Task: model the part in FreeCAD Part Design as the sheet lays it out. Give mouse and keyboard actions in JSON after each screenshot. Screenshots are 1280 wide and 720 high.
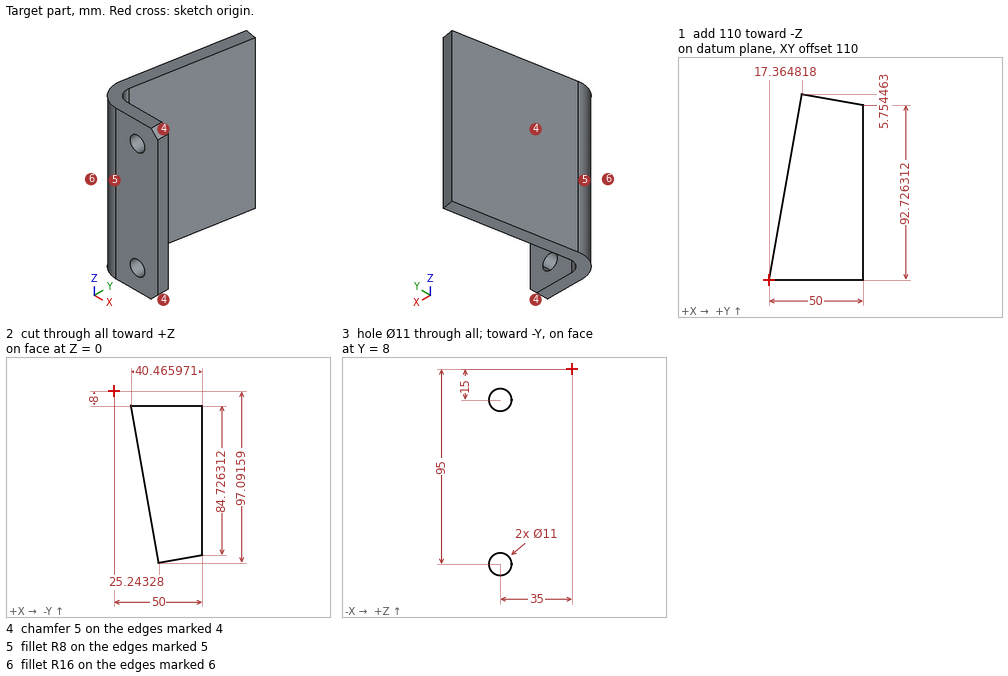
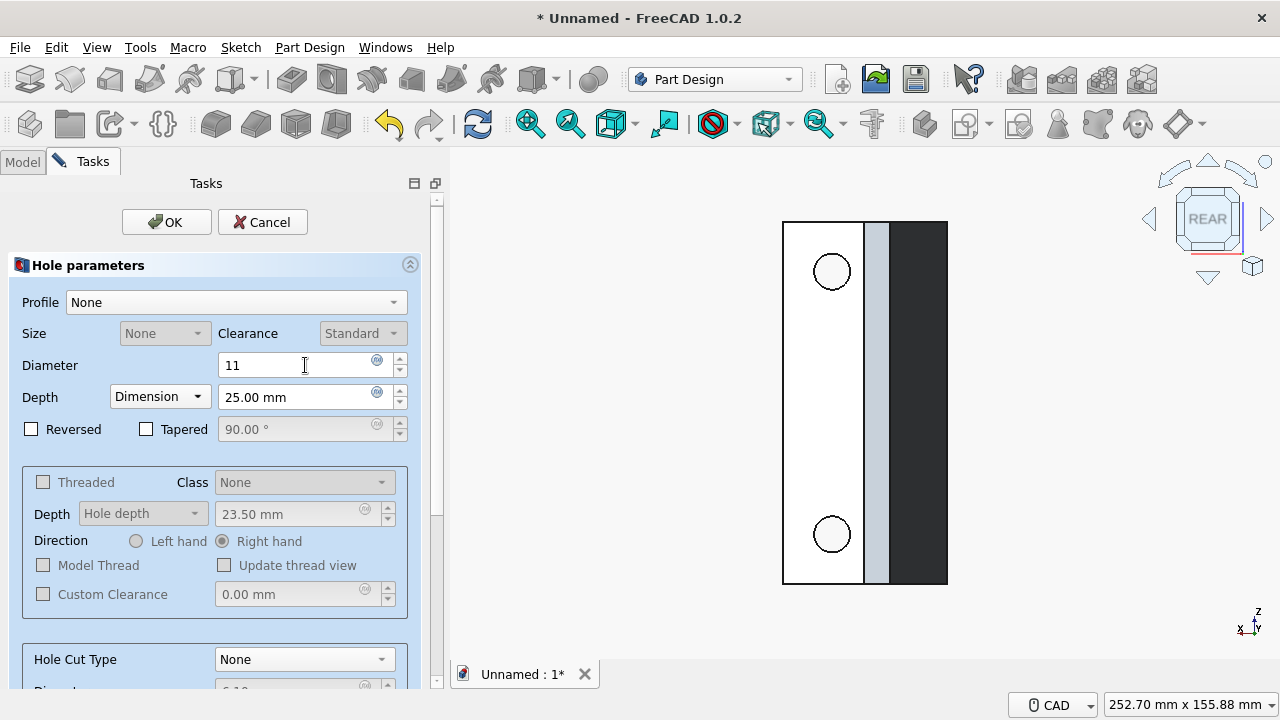
{"action": "left_click", "coordinate": [161, 396]}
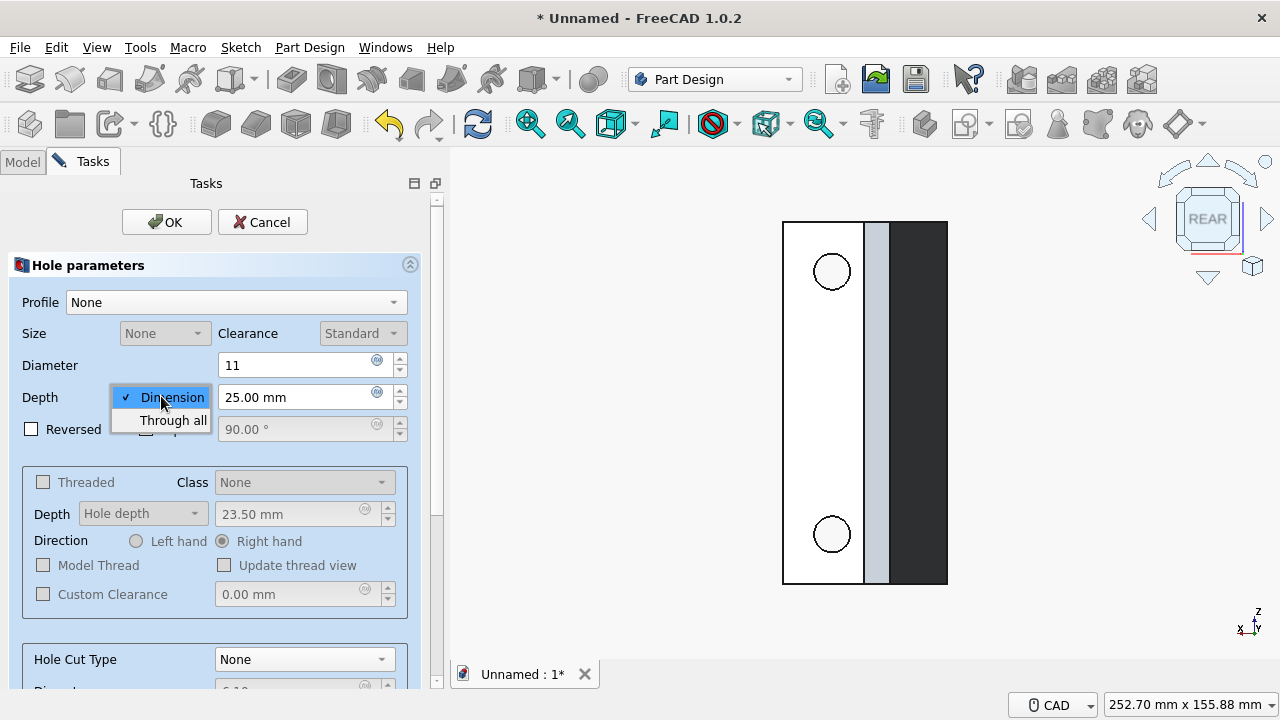
{"action": "left_click", "coordinate": [160, 420]}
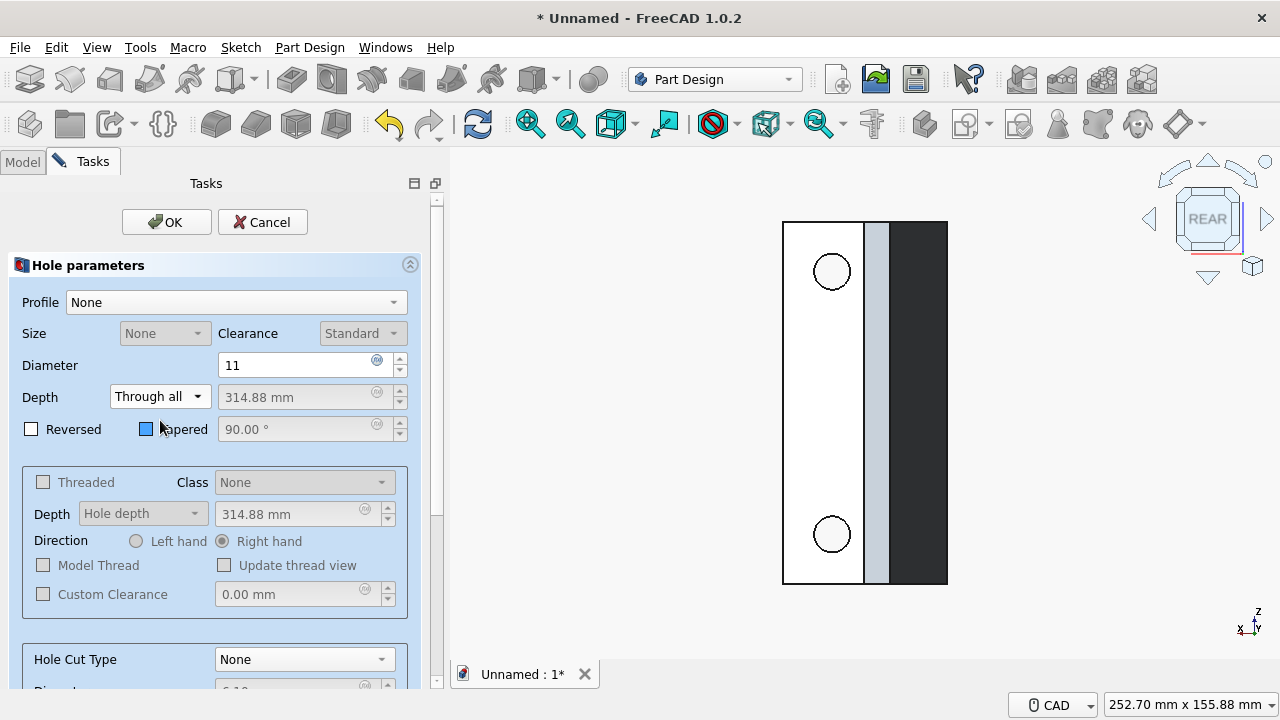
{"action": "left_click", "coordinate": [167, 222]}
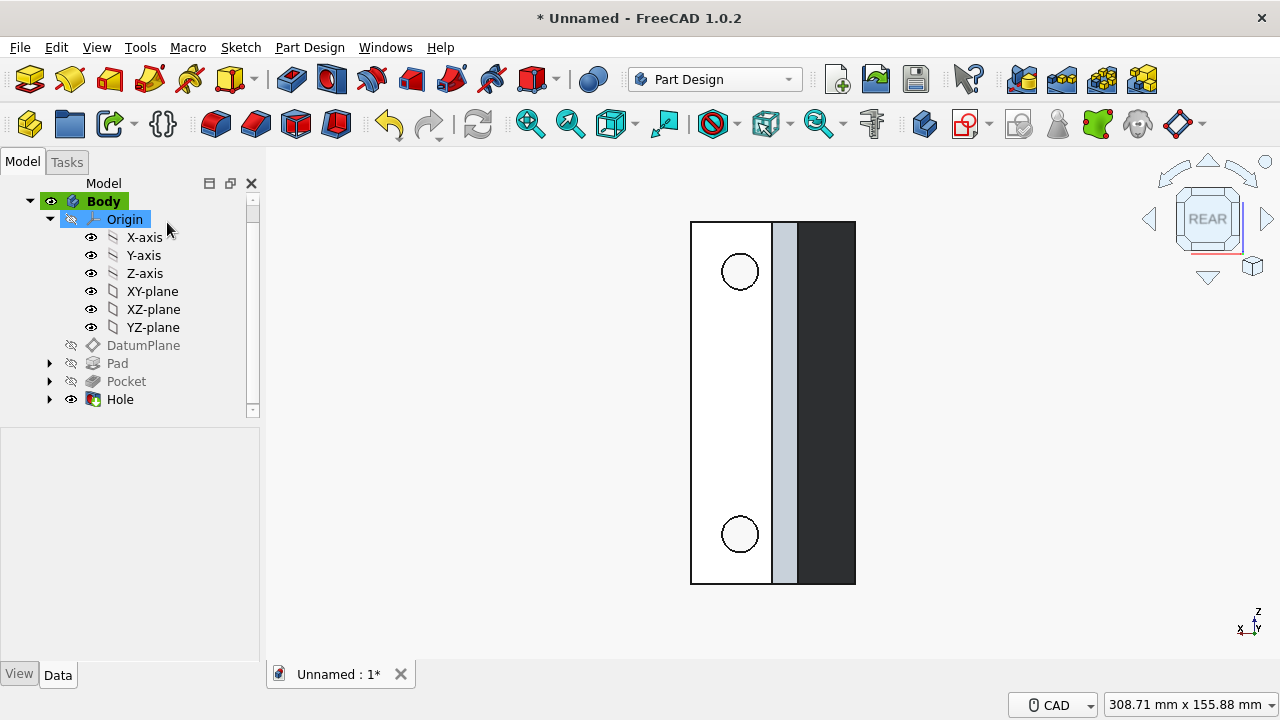
{"action": "key", "text": "0"}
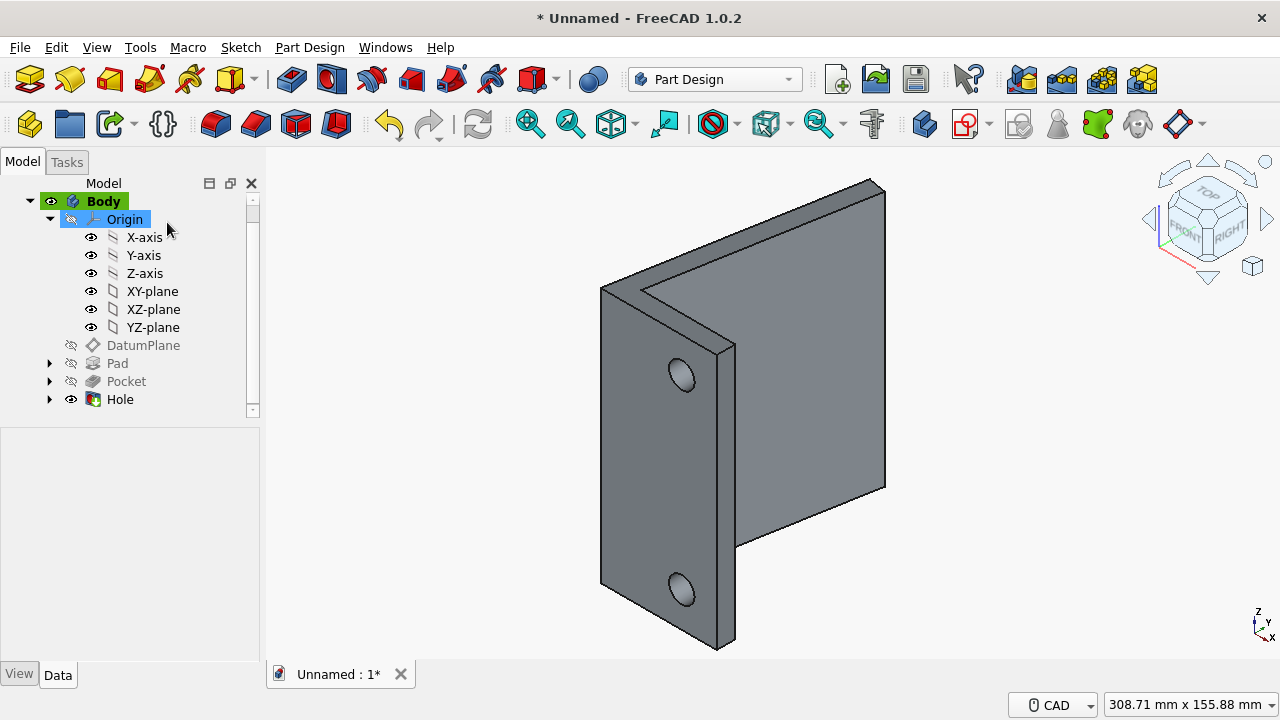
{"action": "left_click", "coordinate": [726, 349]}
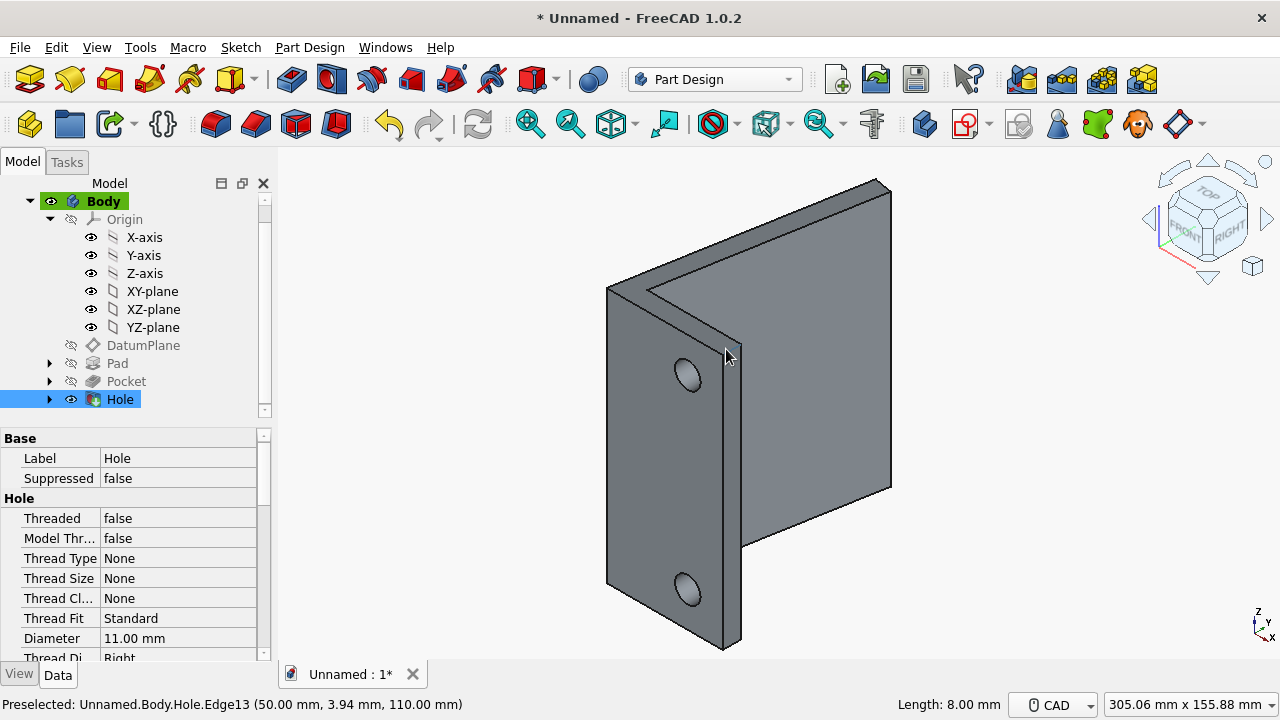
{"action": "key", "text": "2"}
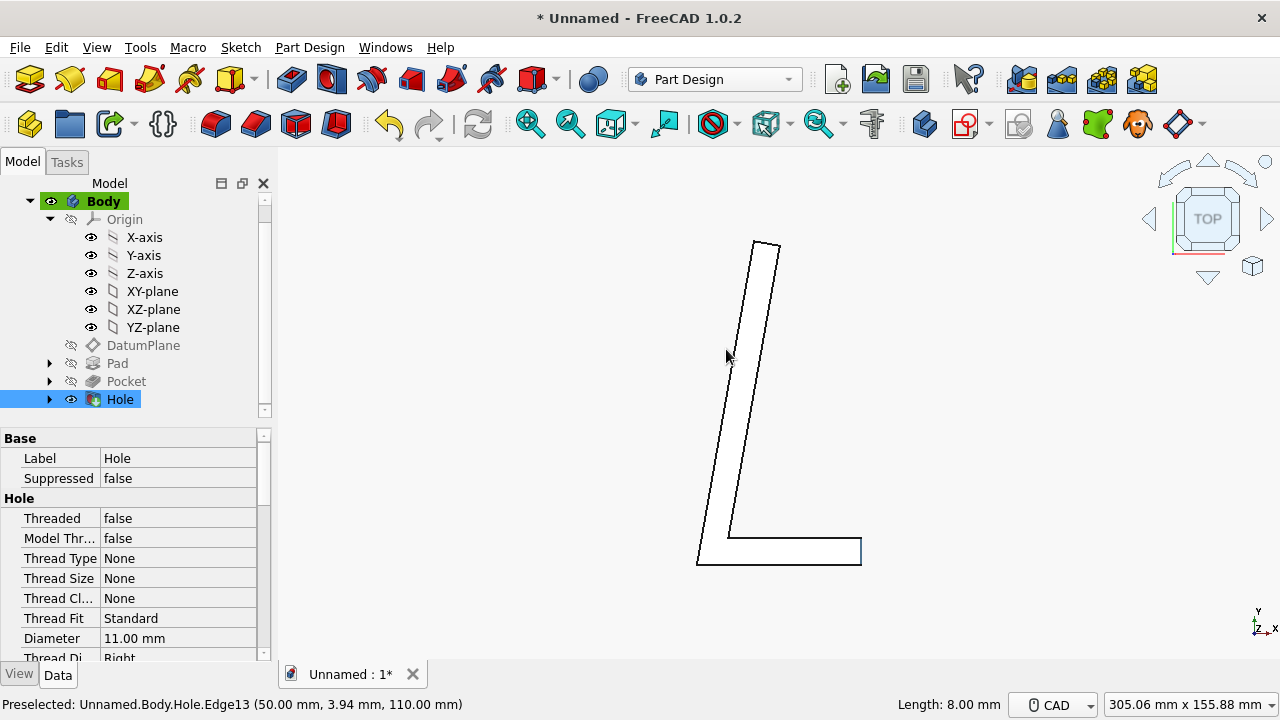
{"action": "key", "text": "1"}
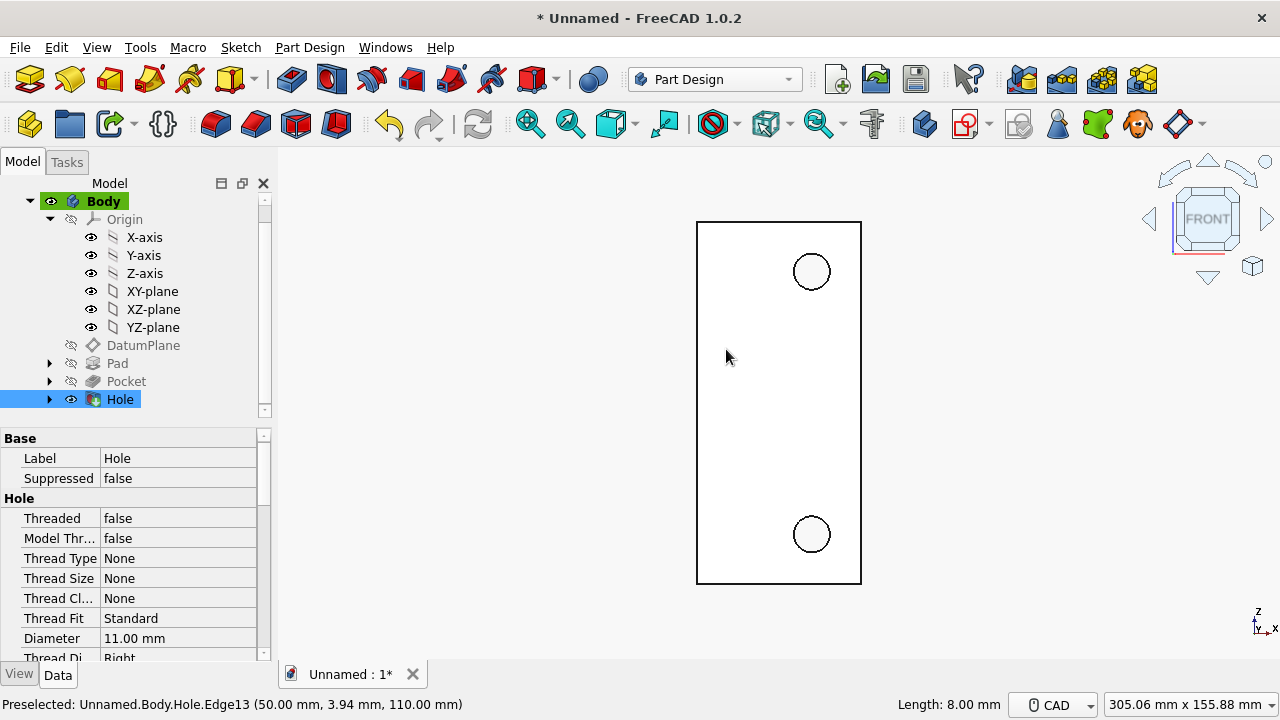
{"action": "key", "text": "3"}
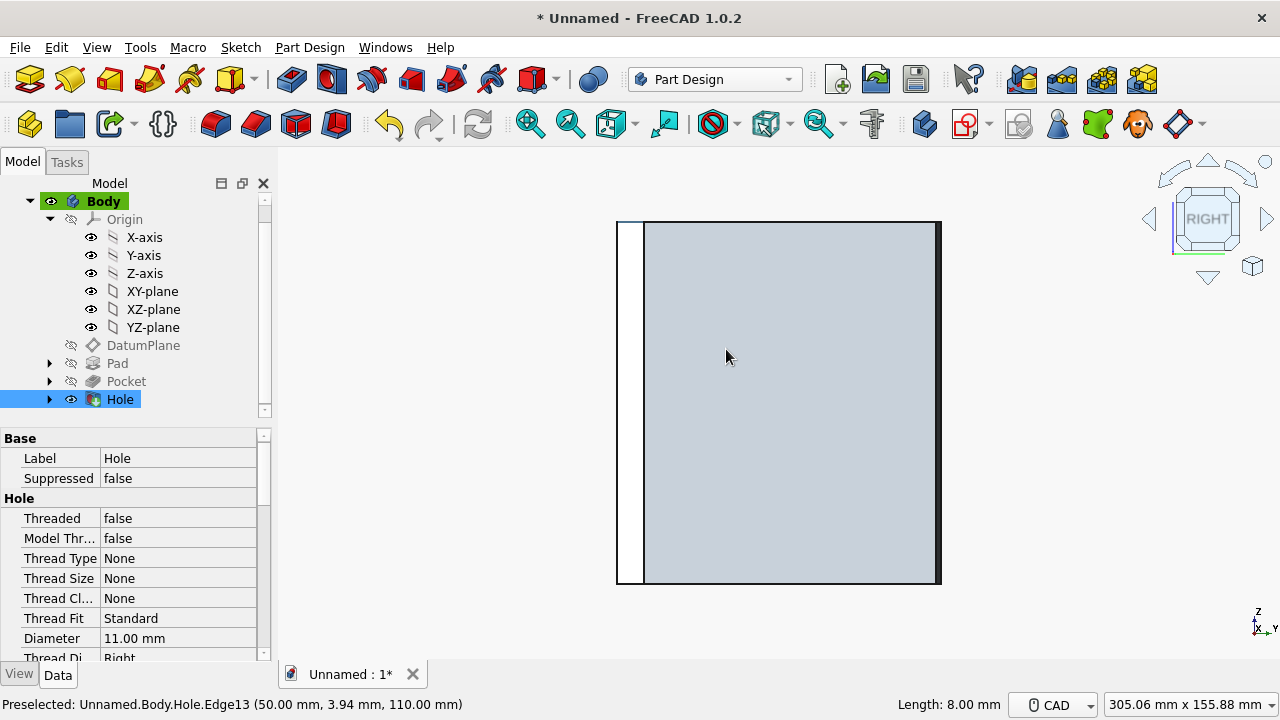
{"action": "left_click", "coordinate": [630, 583], "text": "ctrl"}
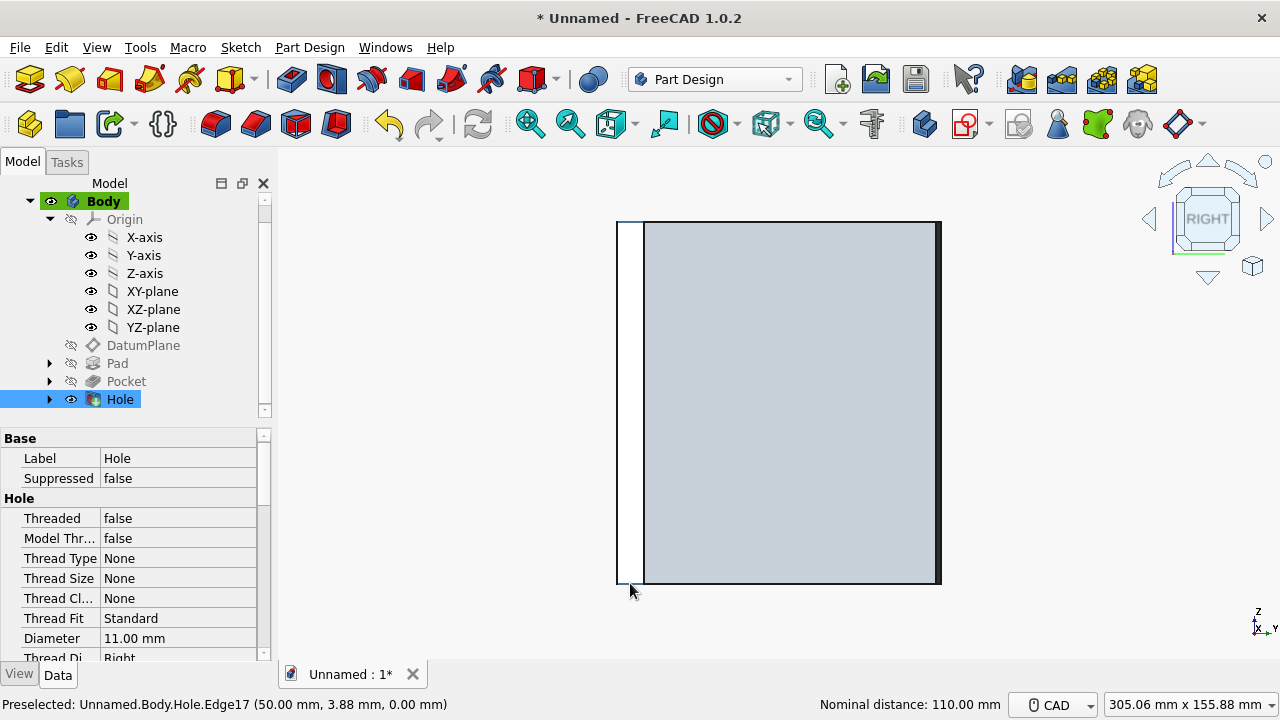
{"action": "left_click", "coordinate": [256, 124]}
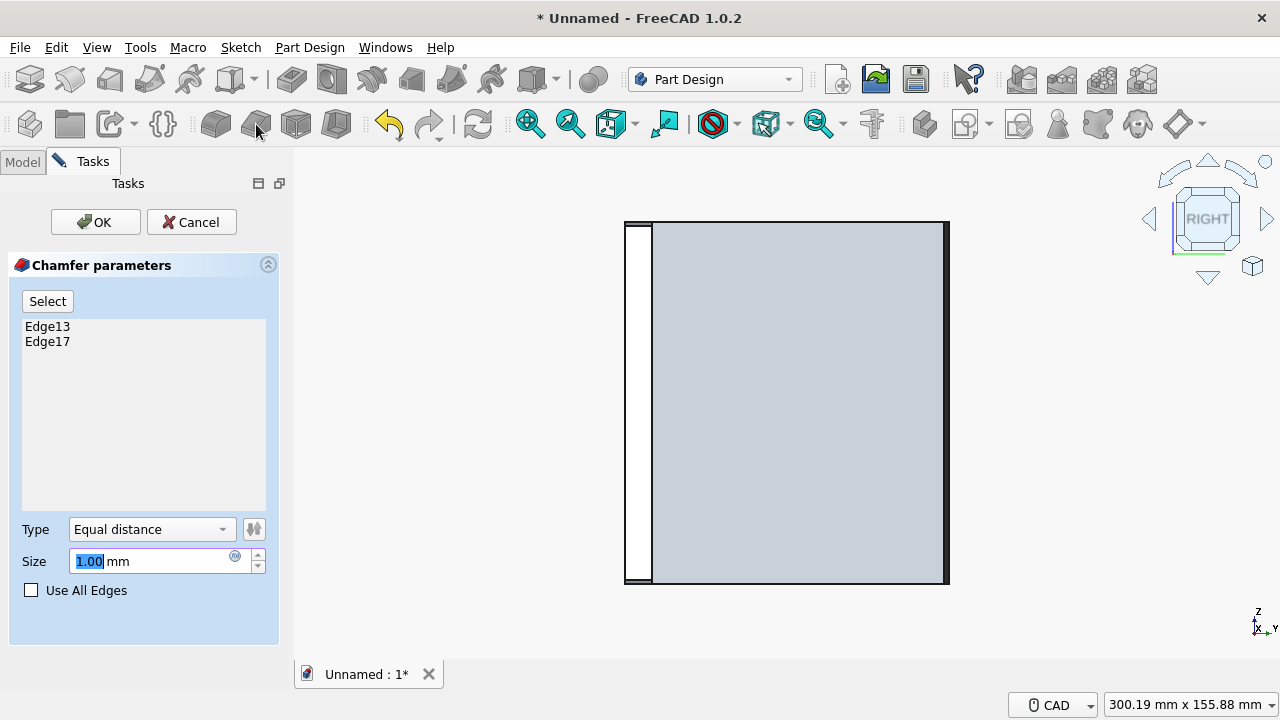
{"action": "type", "text": "5"}
{"action": "key", "text": "Tab"}